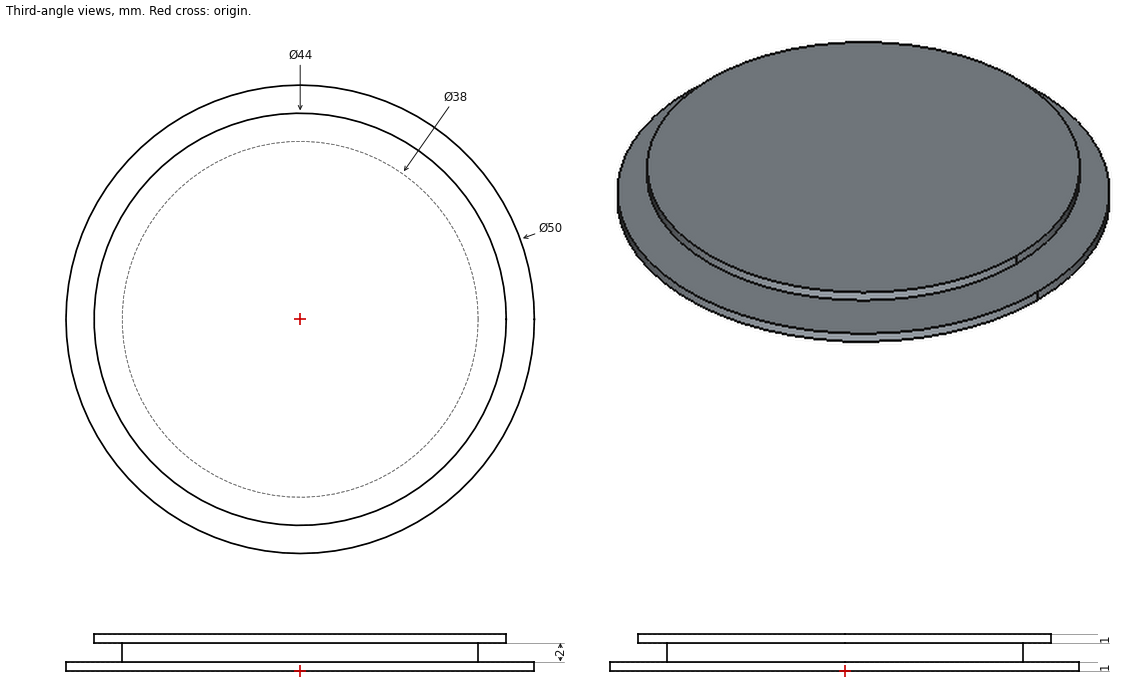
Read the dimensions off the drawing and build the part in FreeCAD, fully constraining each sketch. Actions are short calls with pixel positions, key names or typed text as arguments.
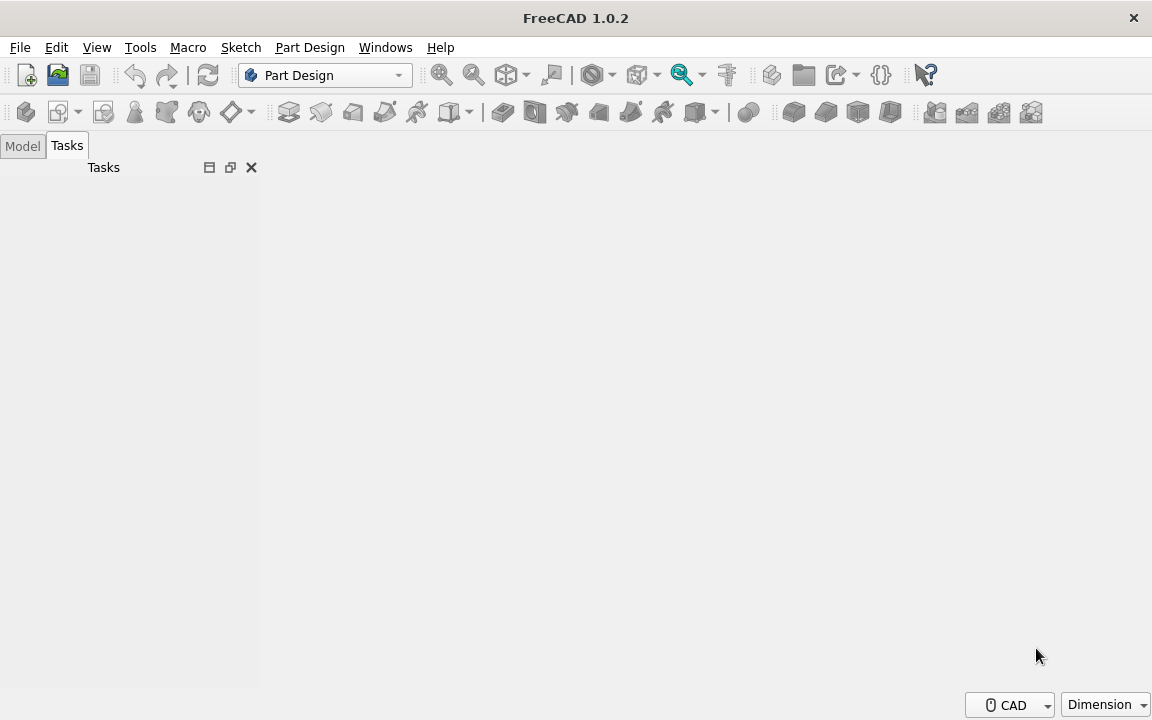
click(26, 76)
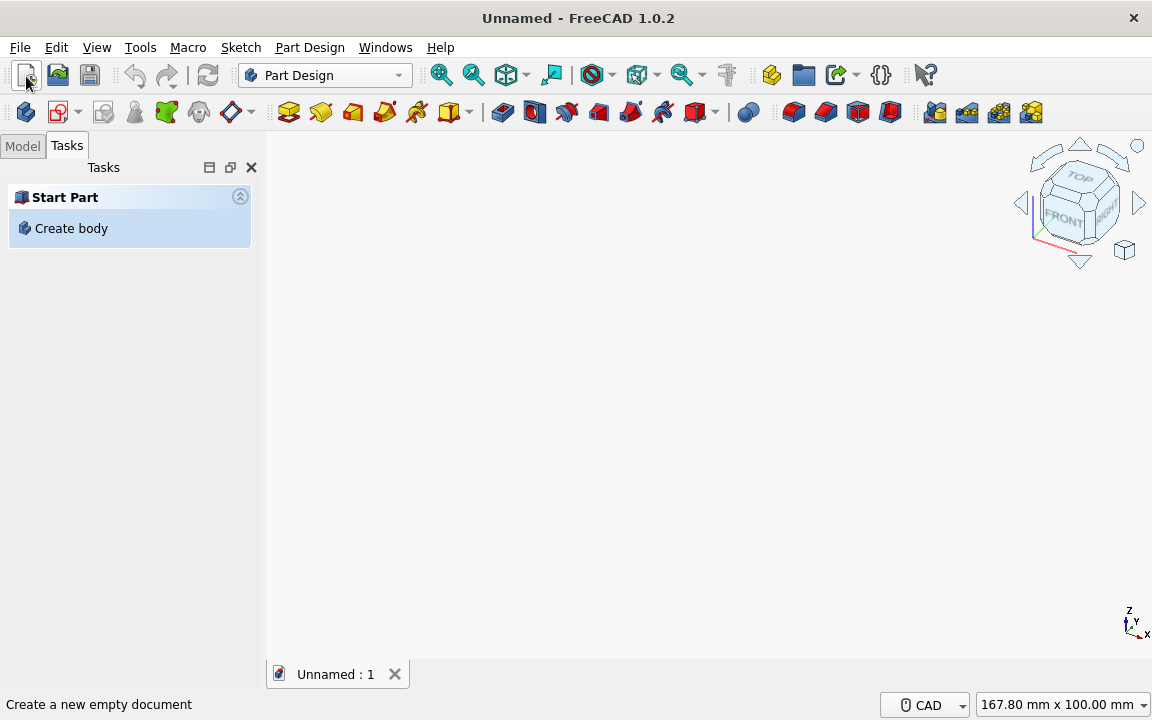
click(58, 112)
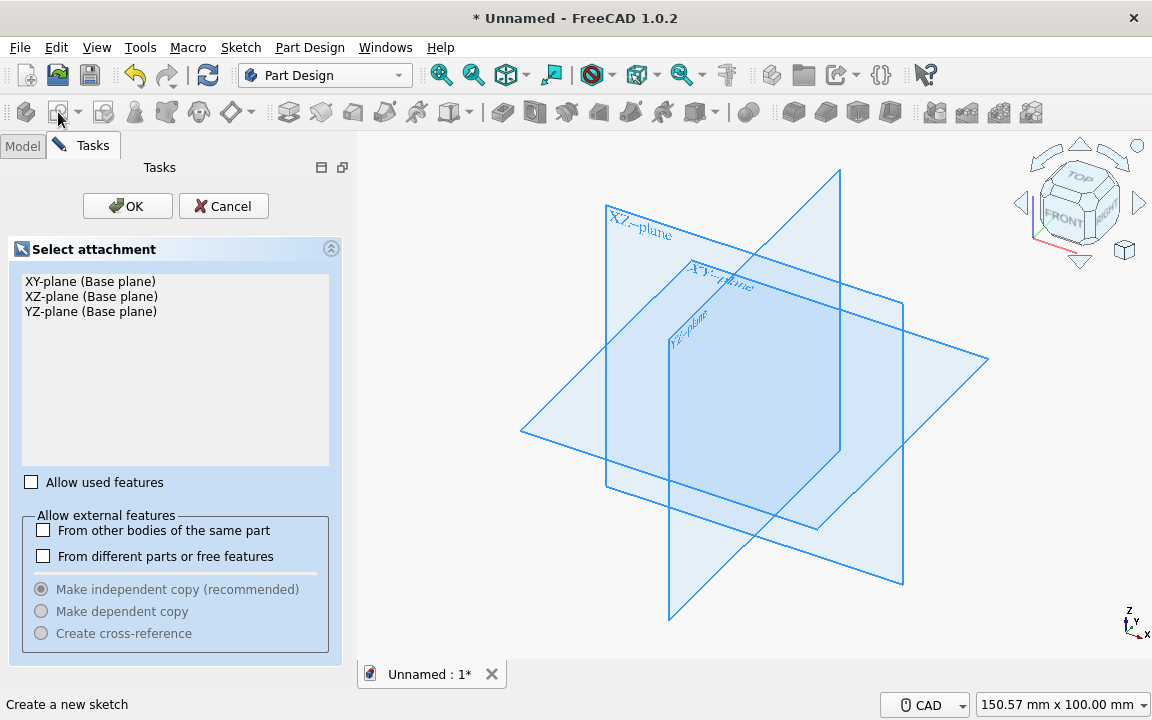
click(82, 282)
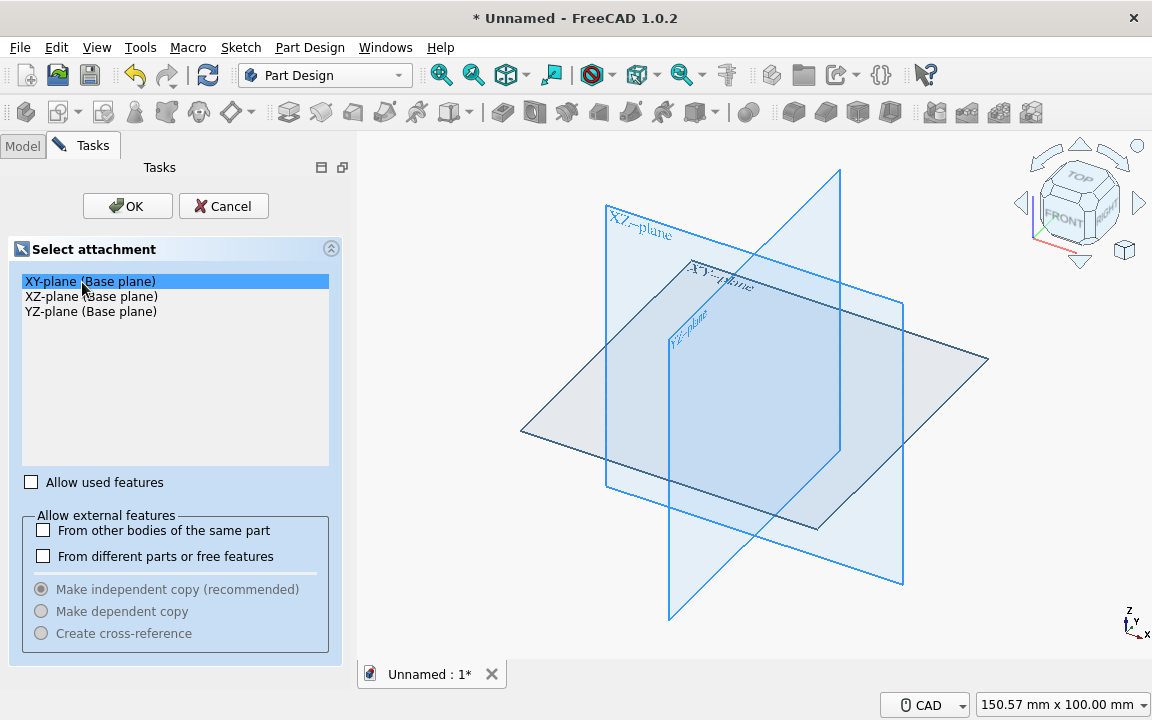
click(128, 206)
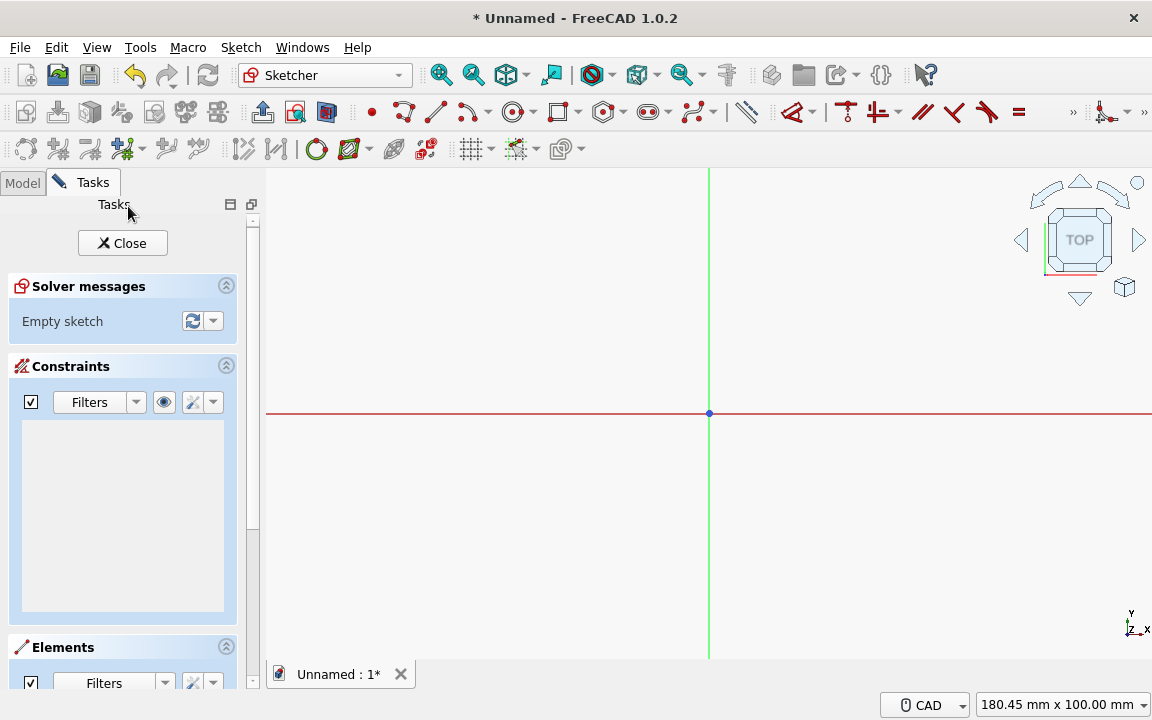
click(514, 112)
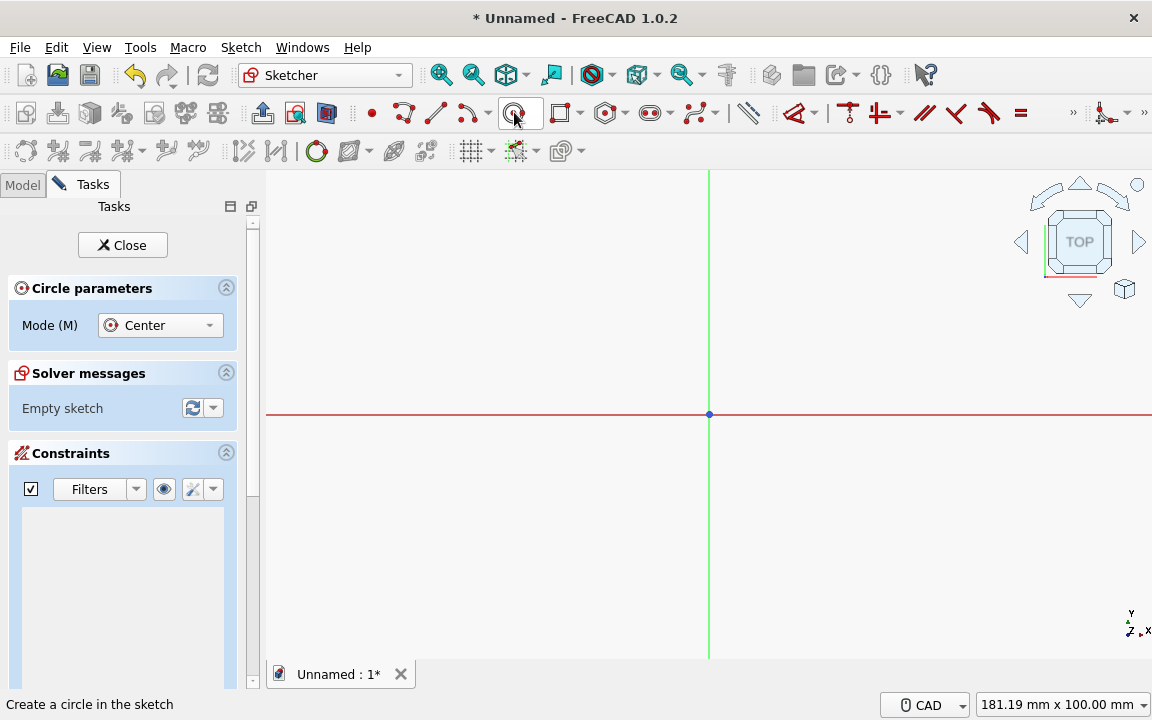
click(709, 414)
move(795, 328)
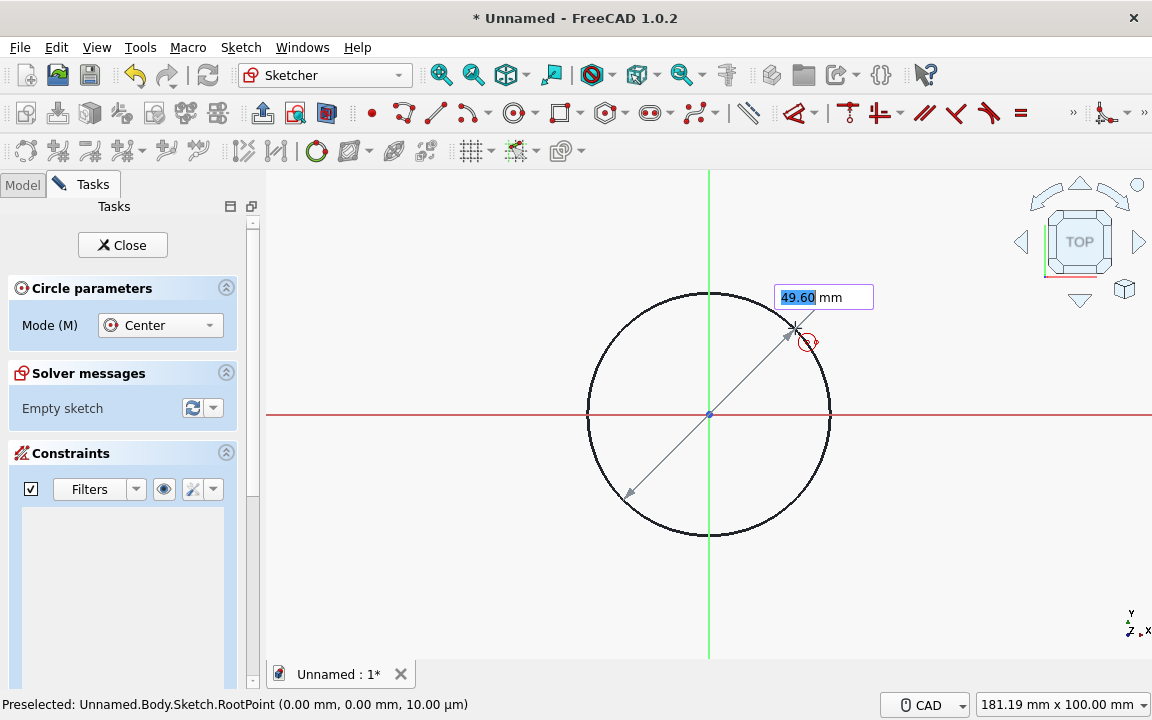
text(50)
key(Return)
key(Escape)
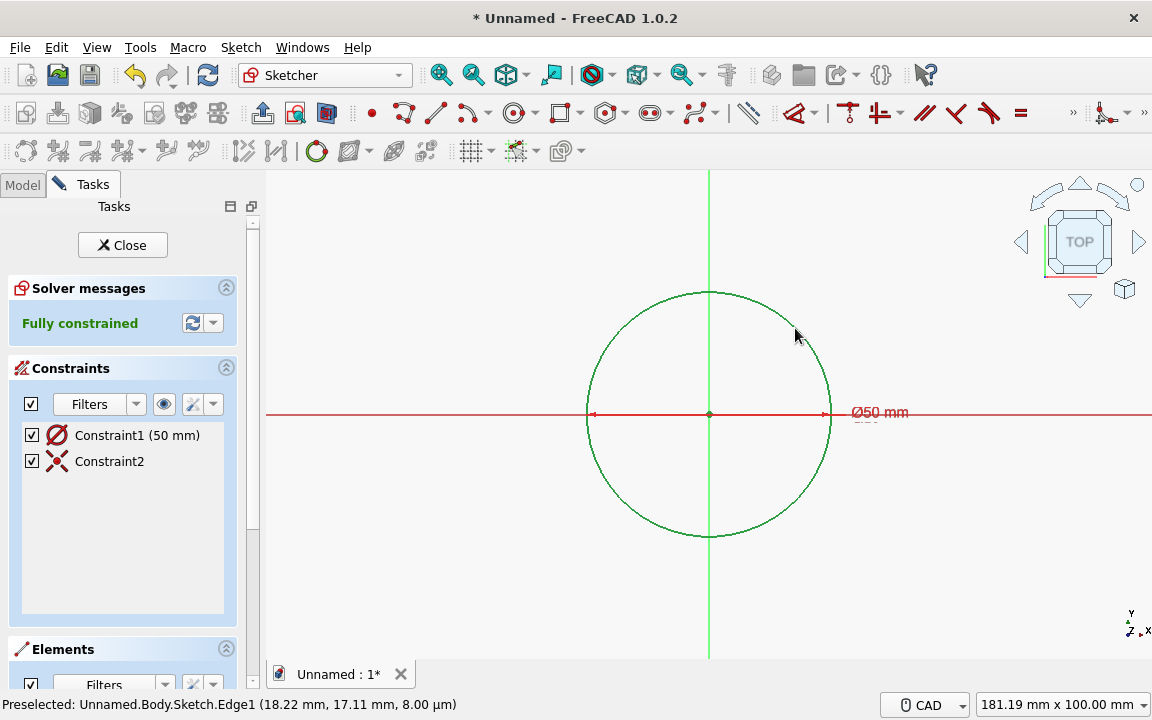
click(123, 245)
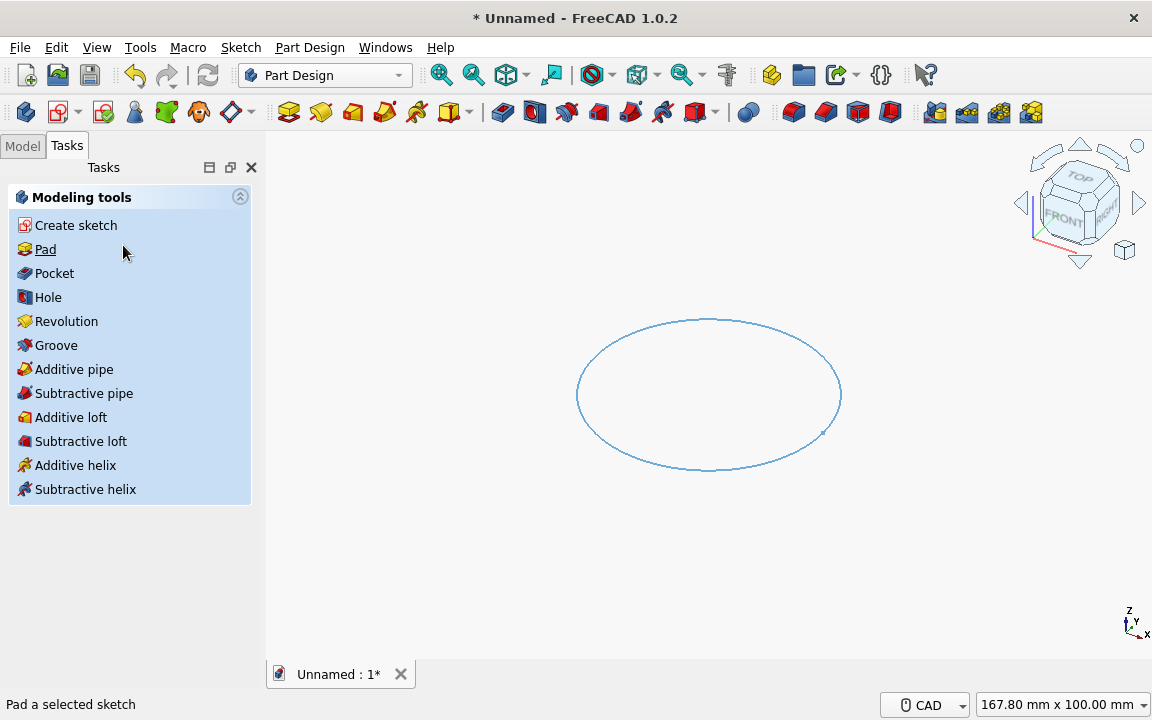
click(290, 112)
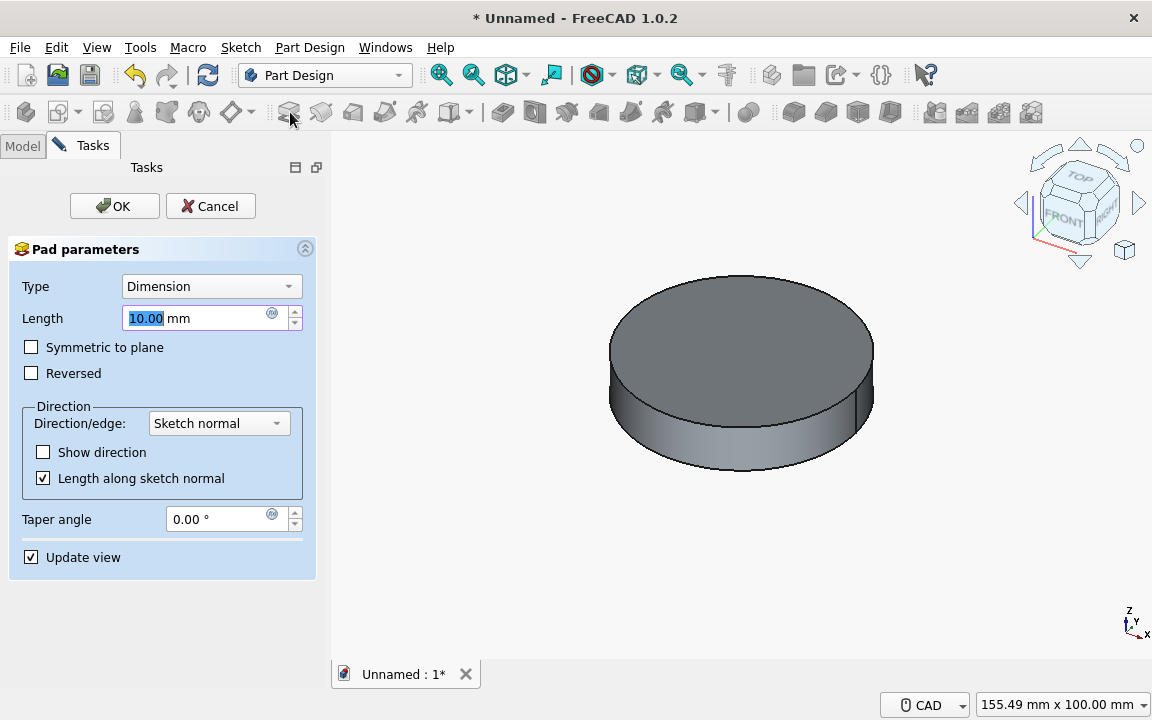
text(1)
key(Tab)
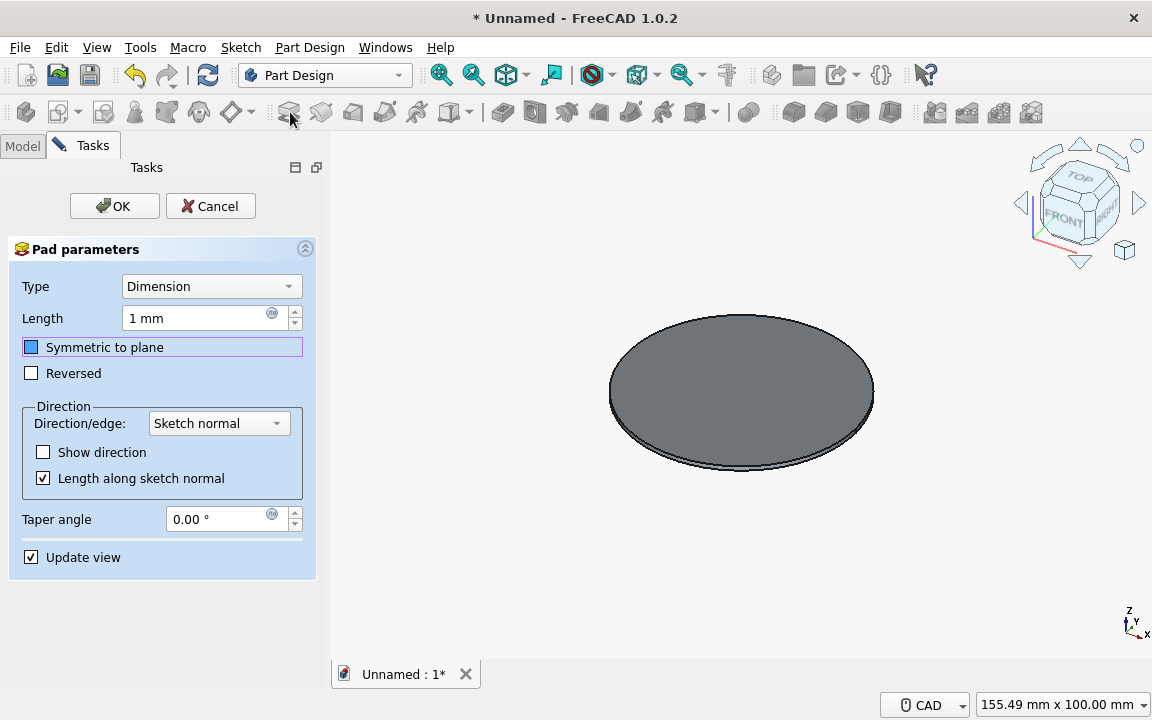
click(115, 206)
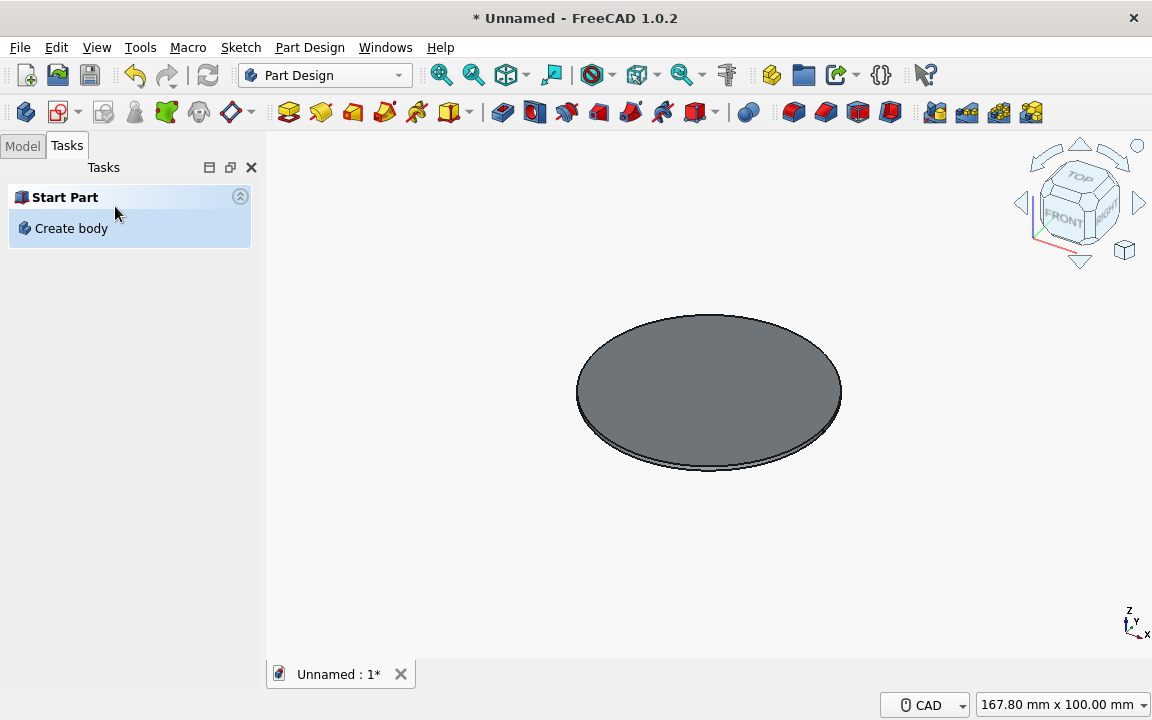
click(442, 76)